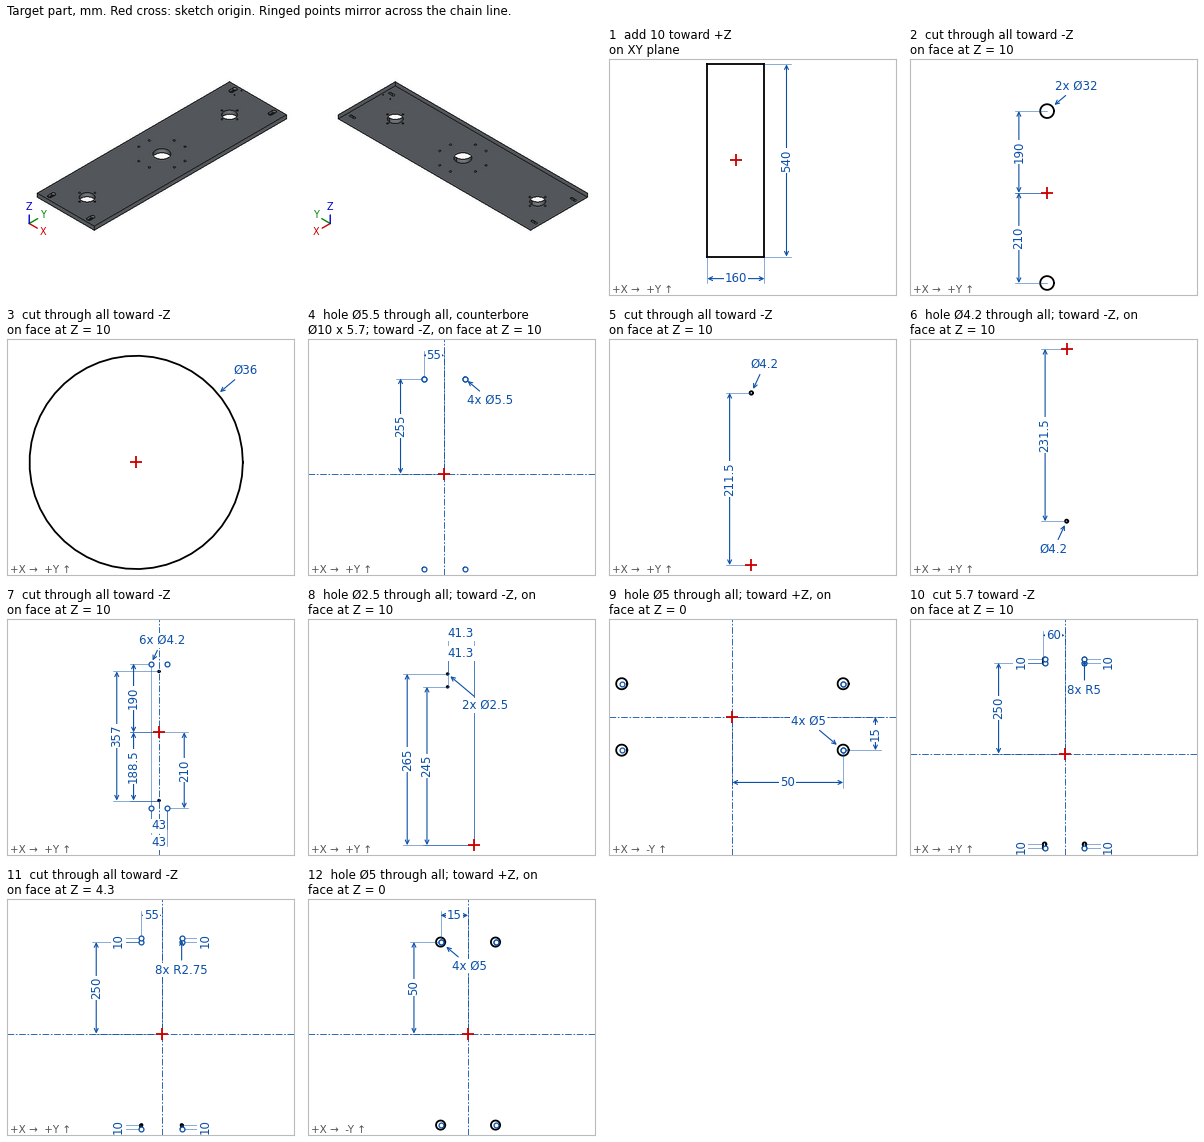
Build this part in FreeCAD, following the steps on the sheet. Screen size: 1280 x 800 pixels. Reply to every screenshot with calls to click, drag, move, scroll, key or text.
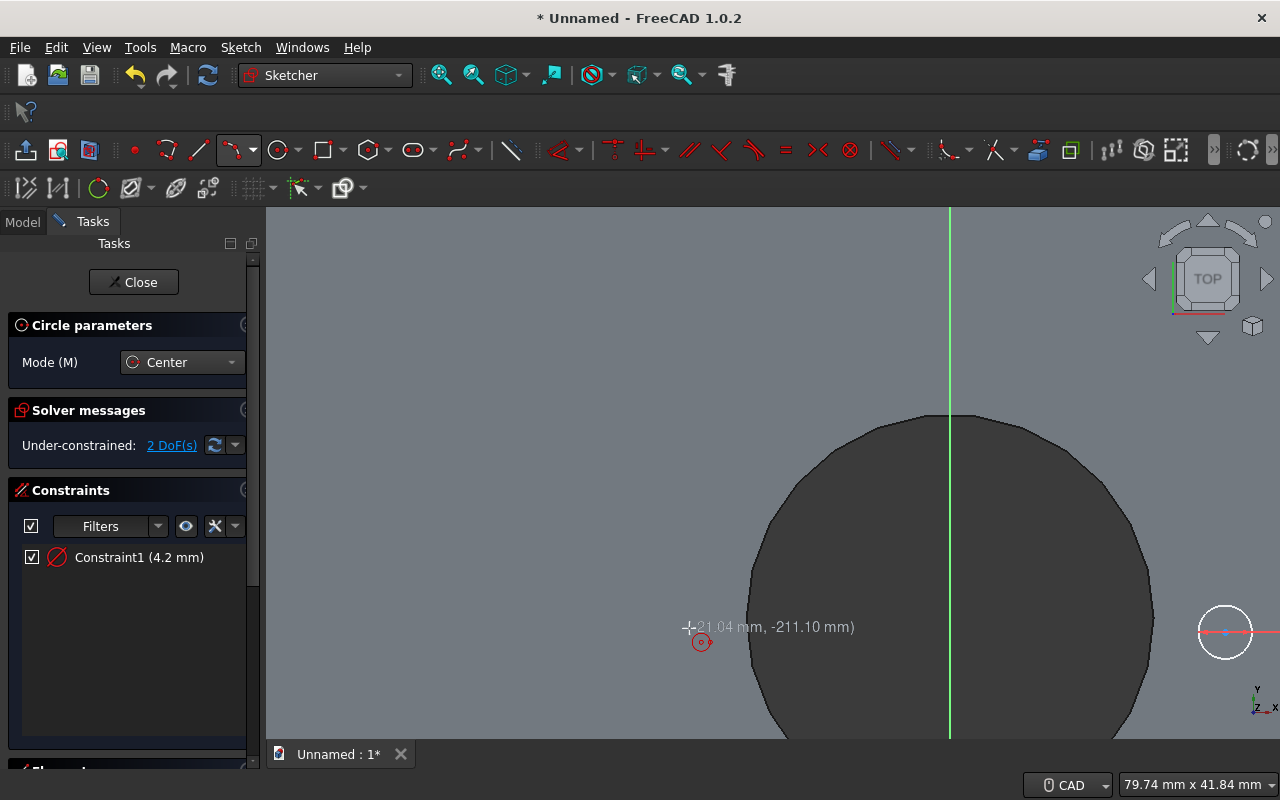
scroll(689, 628, down, 14)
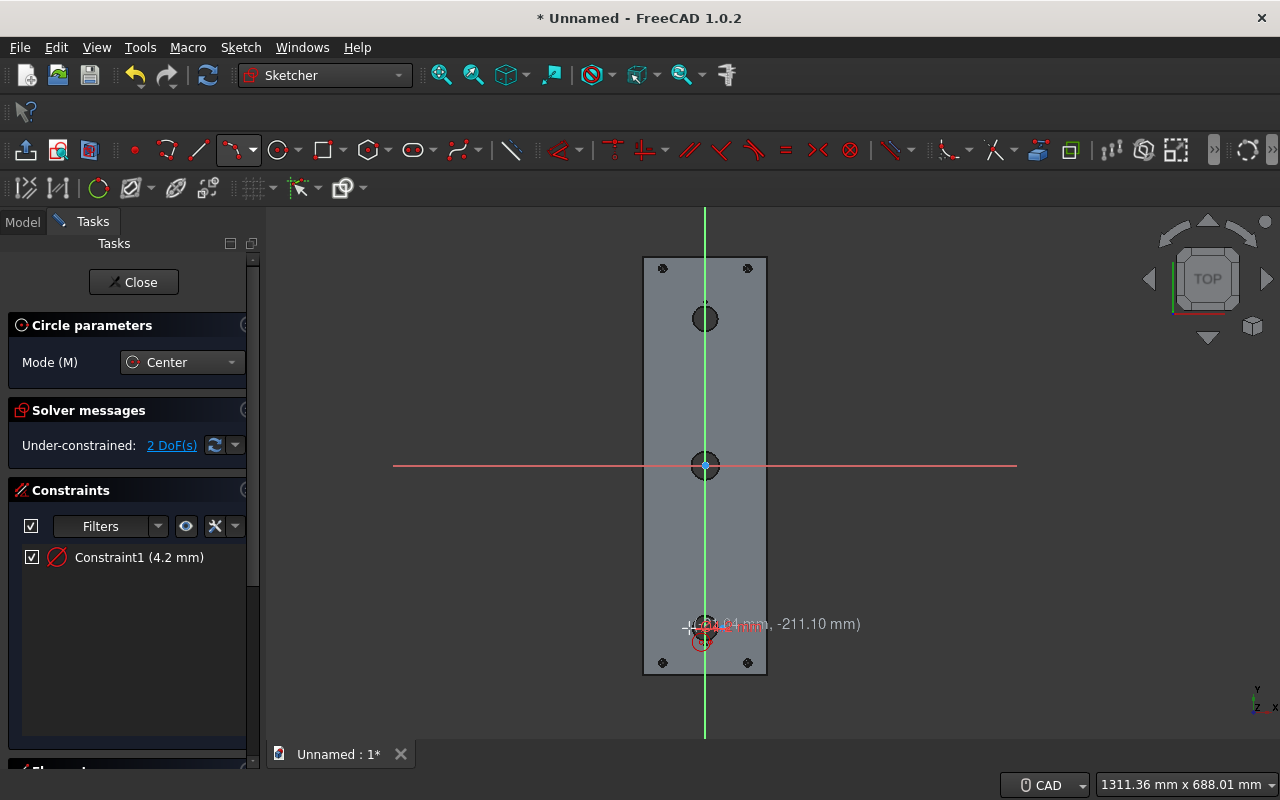
click(689, 628)
move(690, 627)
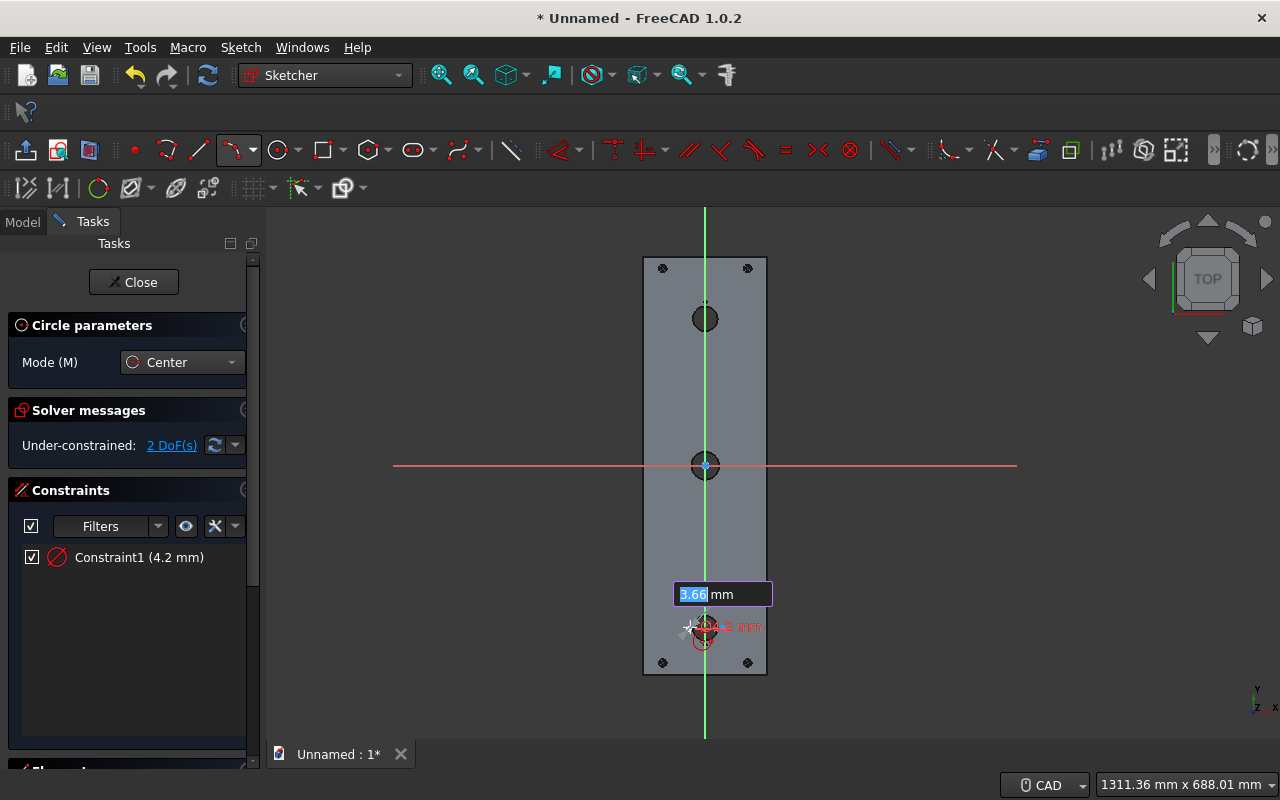
text(4.2)
key(Return)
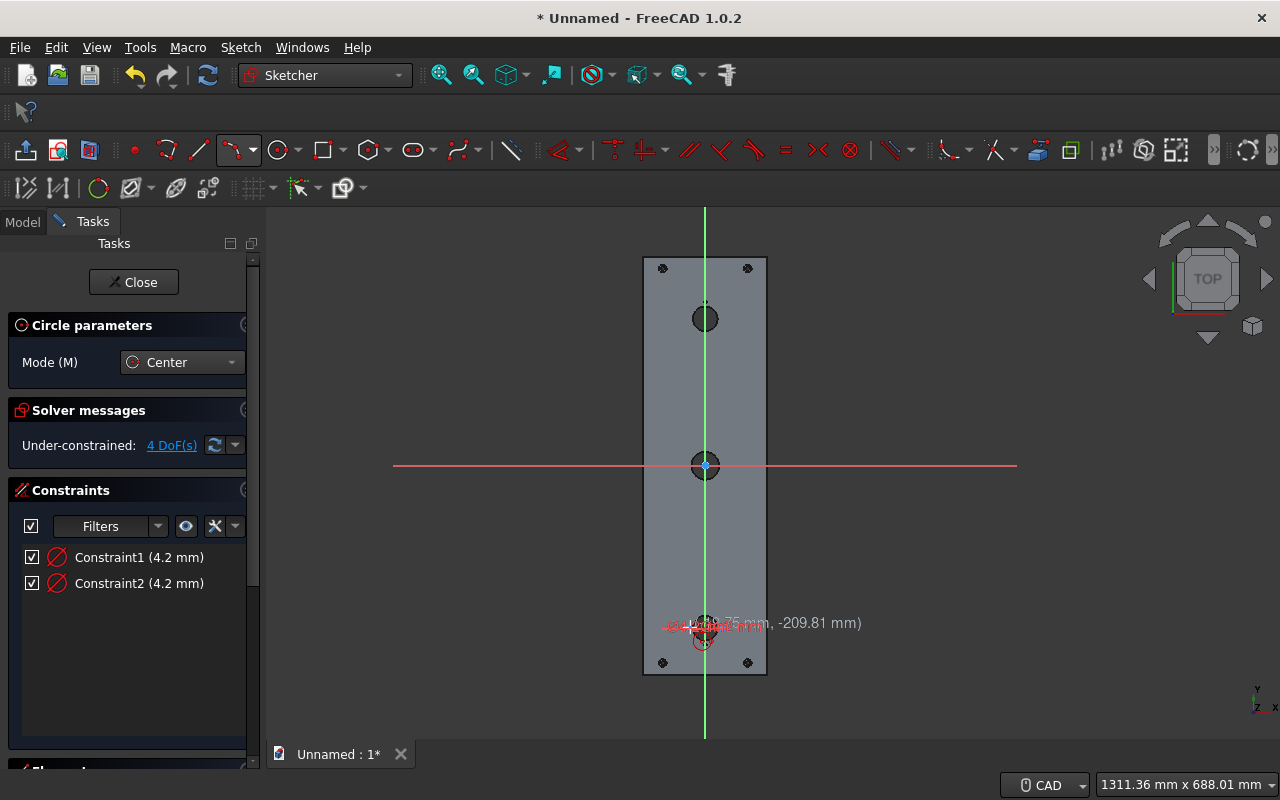
scroll(705, 612, up, 14)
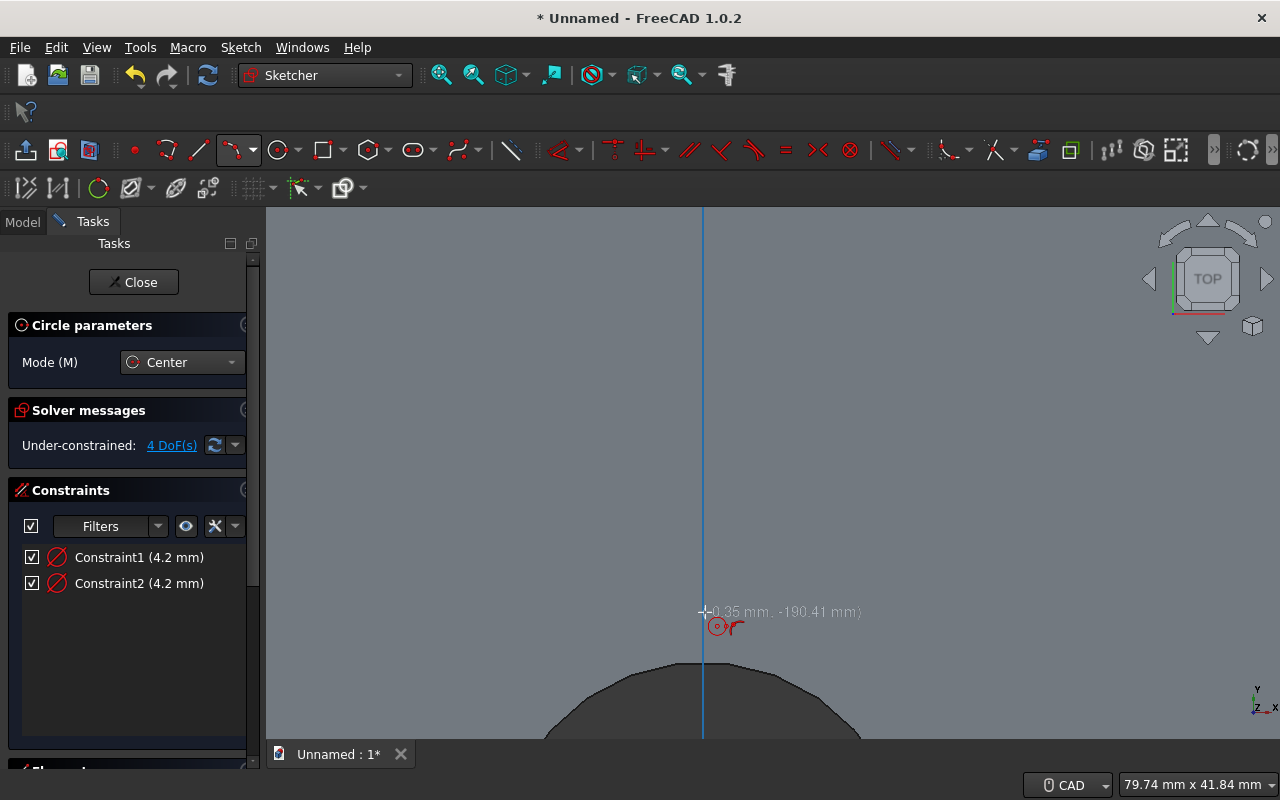
scroll(705, 612, down, 14)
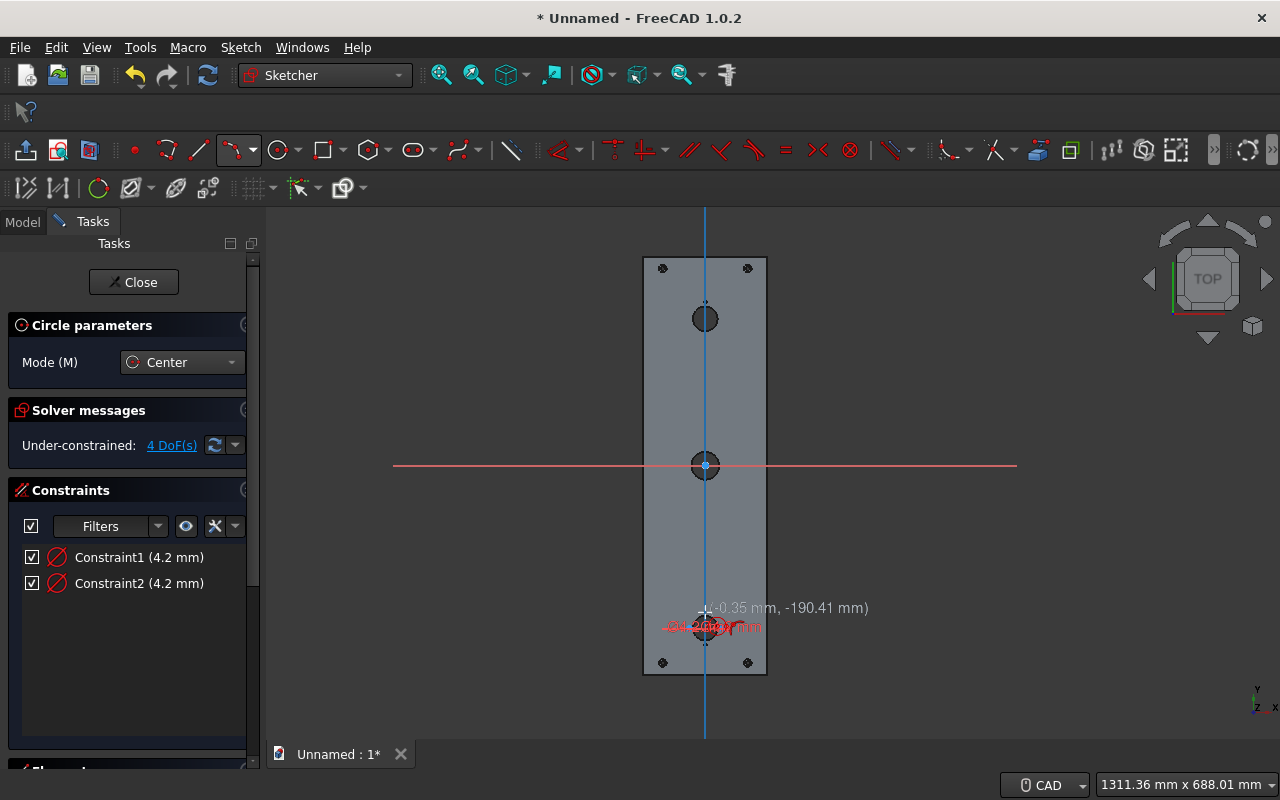
click(705, 612)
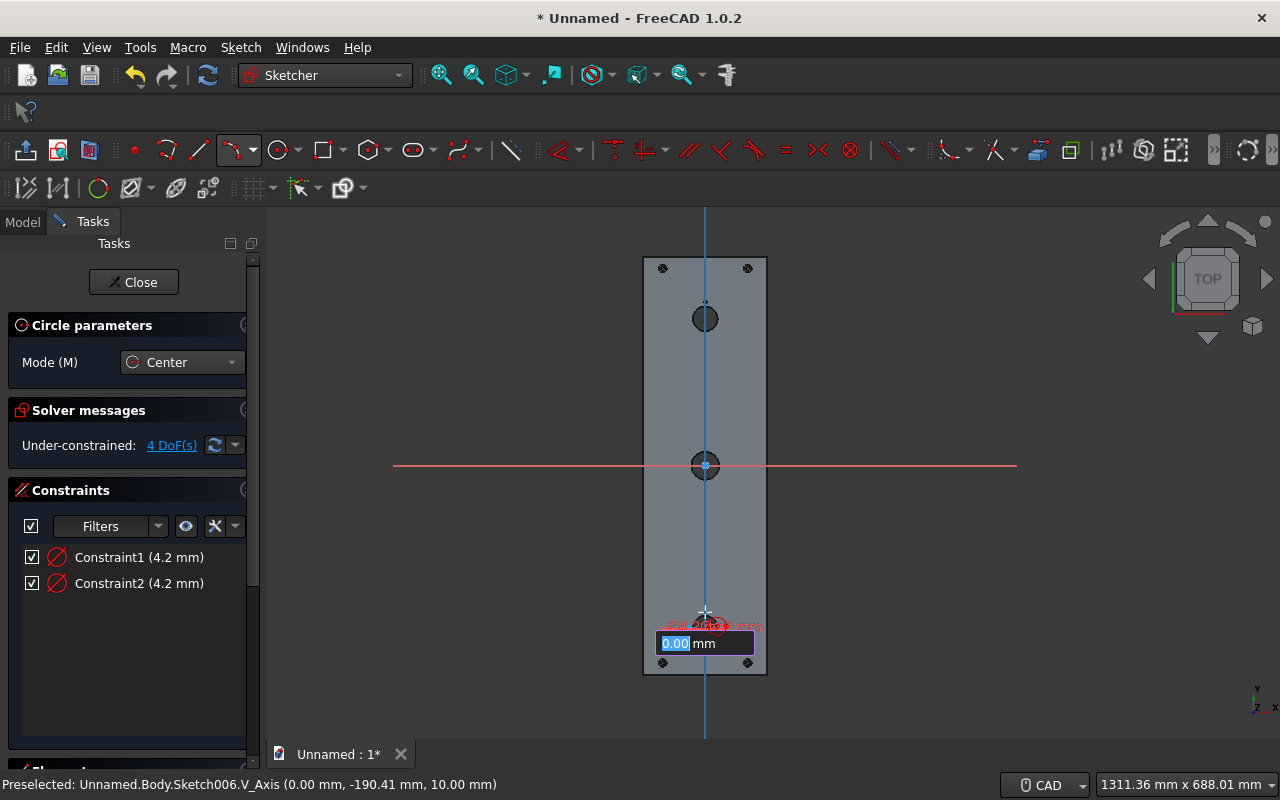
scroll(707, 611, up, 12)
move(700, 603)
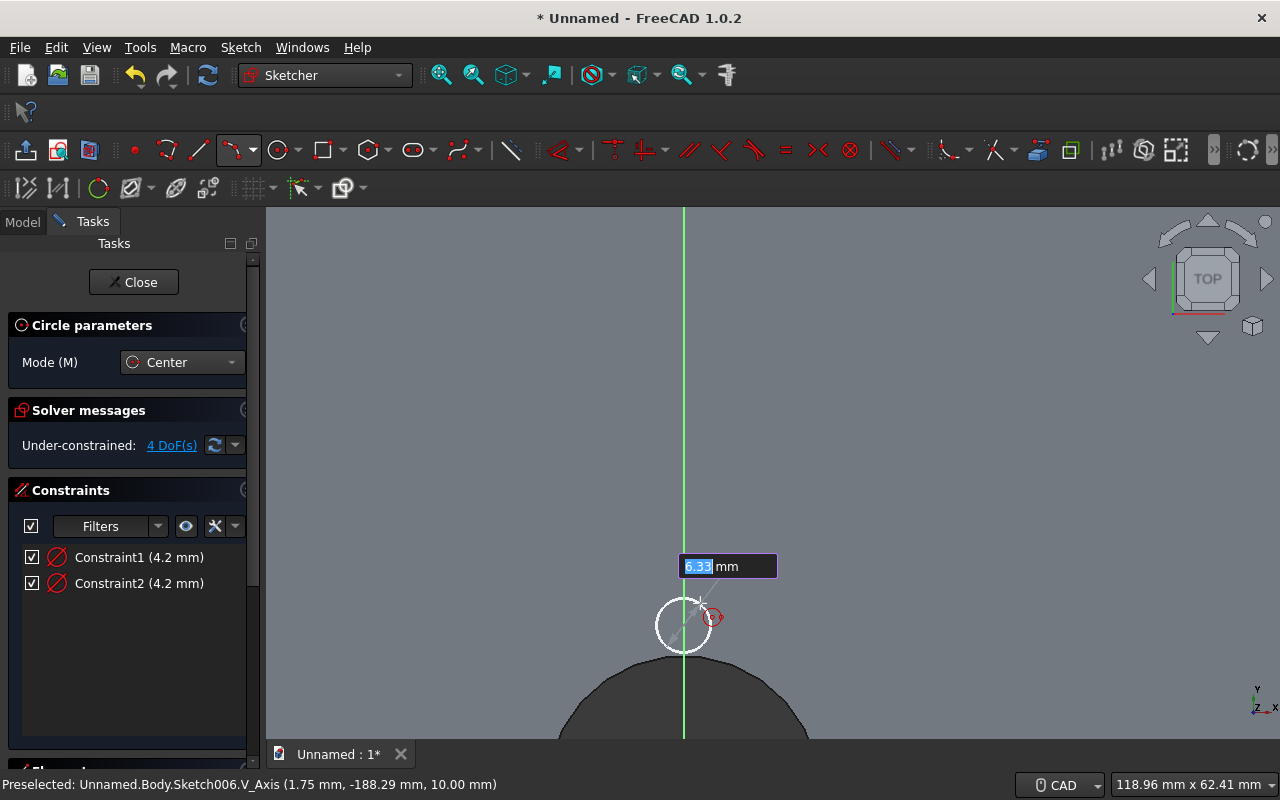
text(4.2)
key(Return)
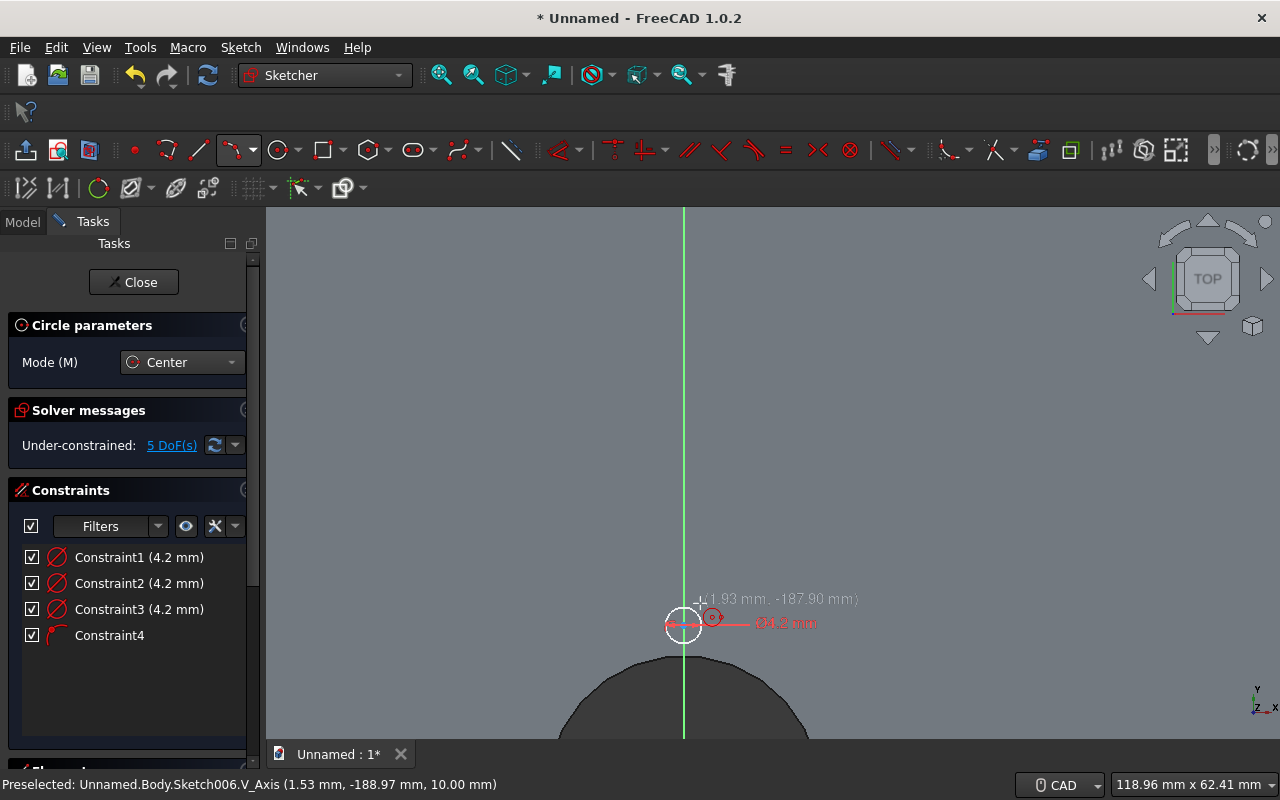
scroll(707, 611, down, 12)